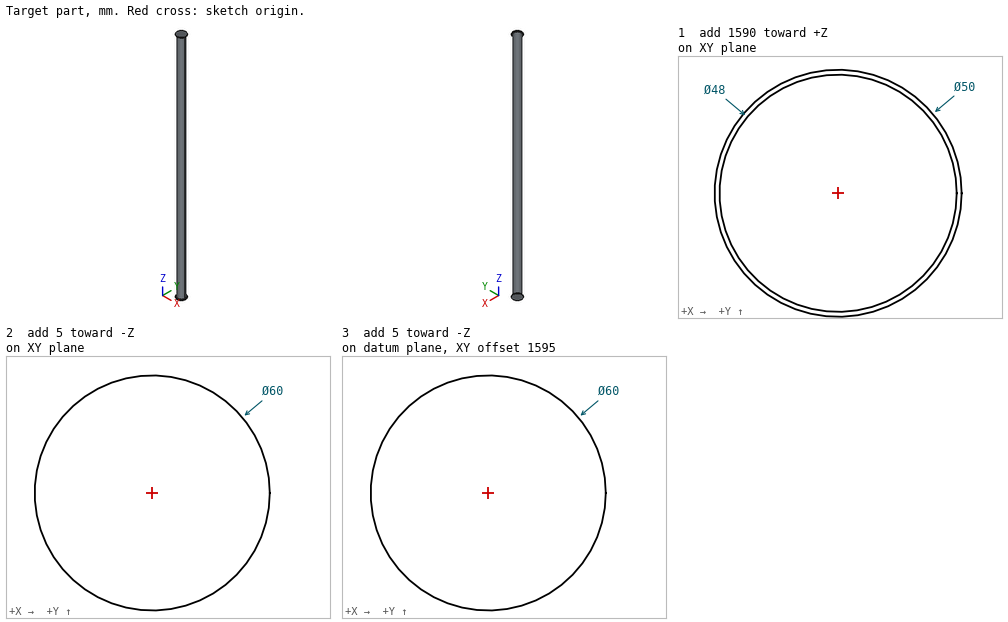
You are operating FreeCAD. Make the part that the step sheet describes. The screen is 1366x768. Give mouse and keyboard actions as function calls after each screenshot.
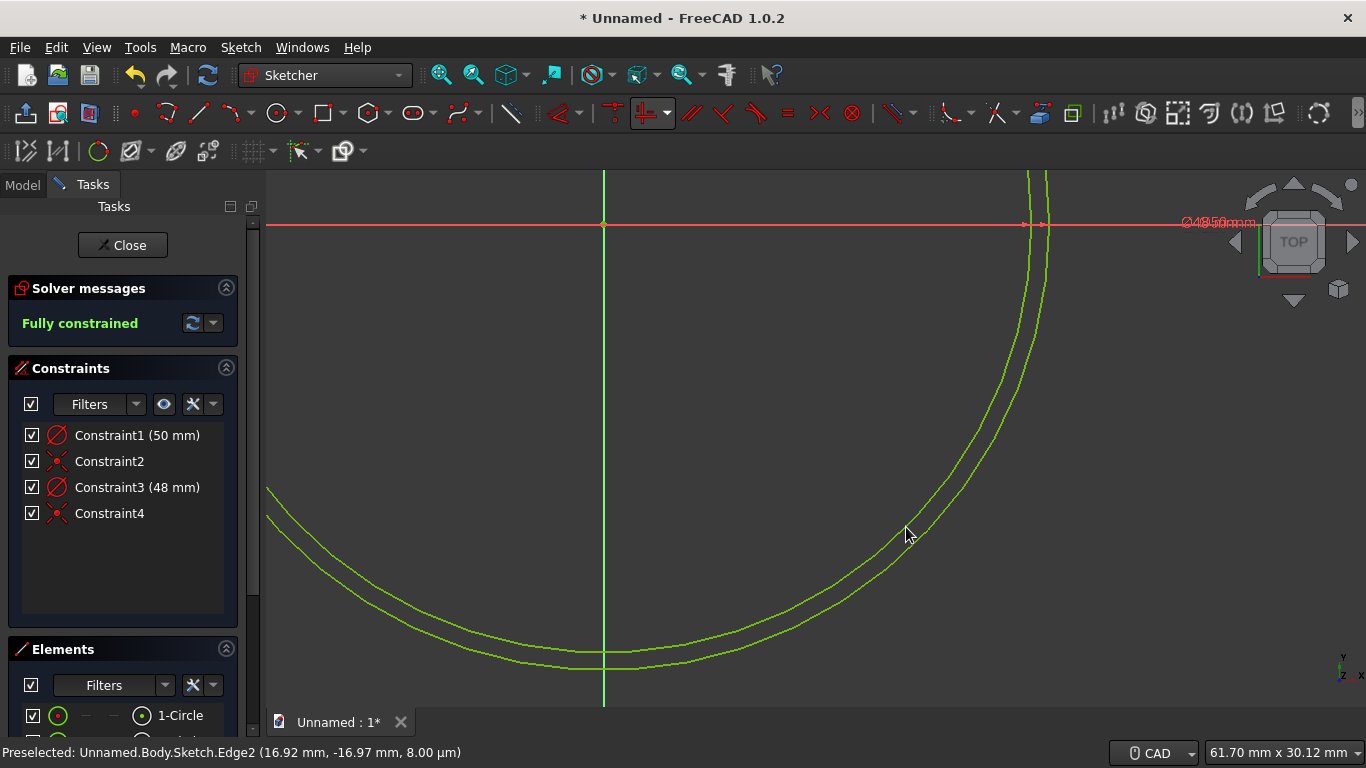
click(123, 245)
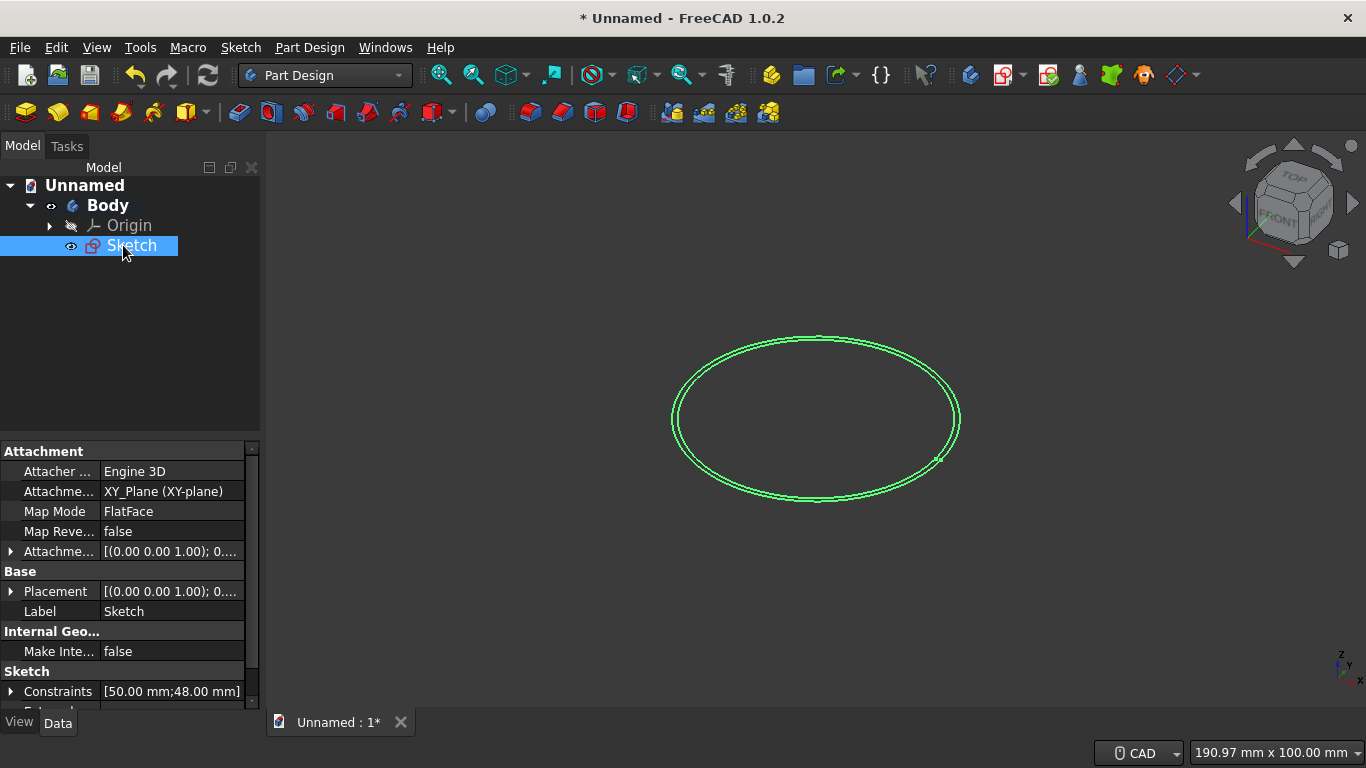
click(26, 112)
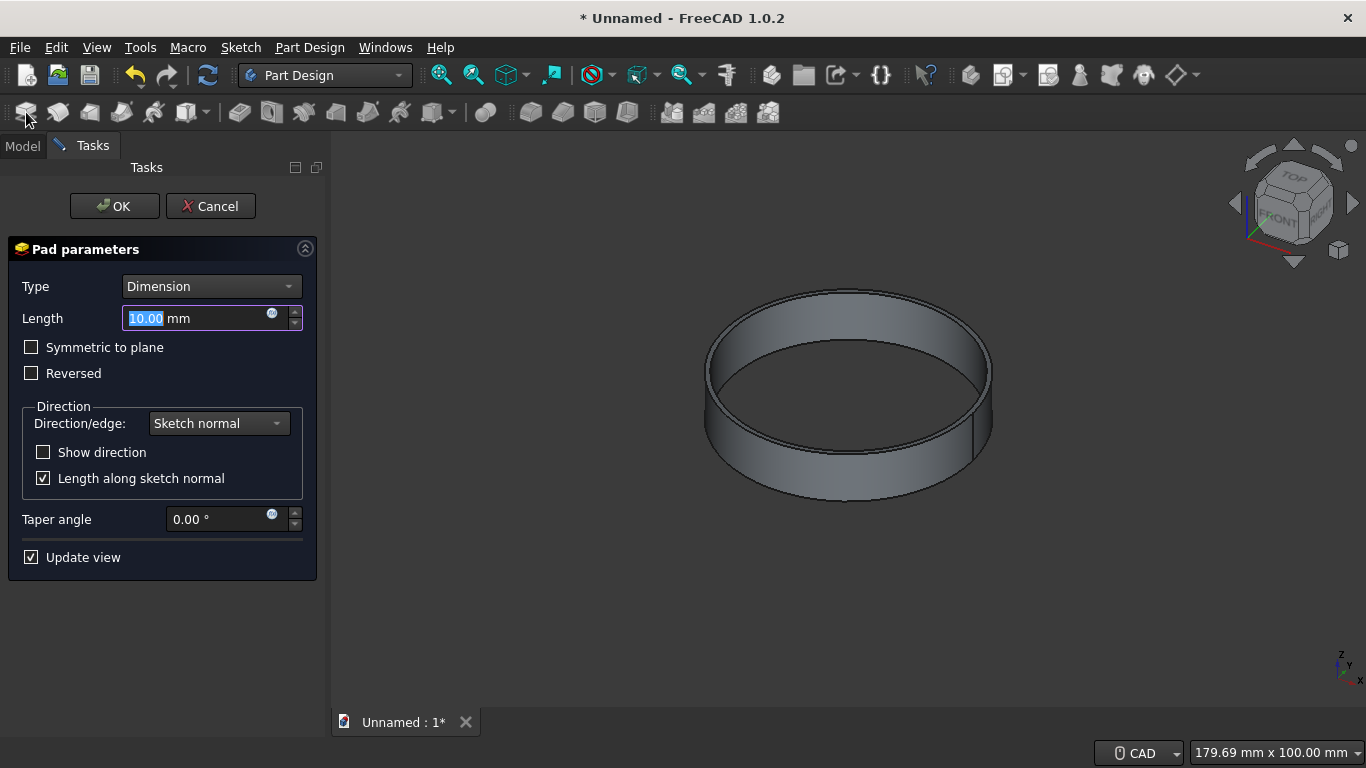
text(1590)
key(Tab)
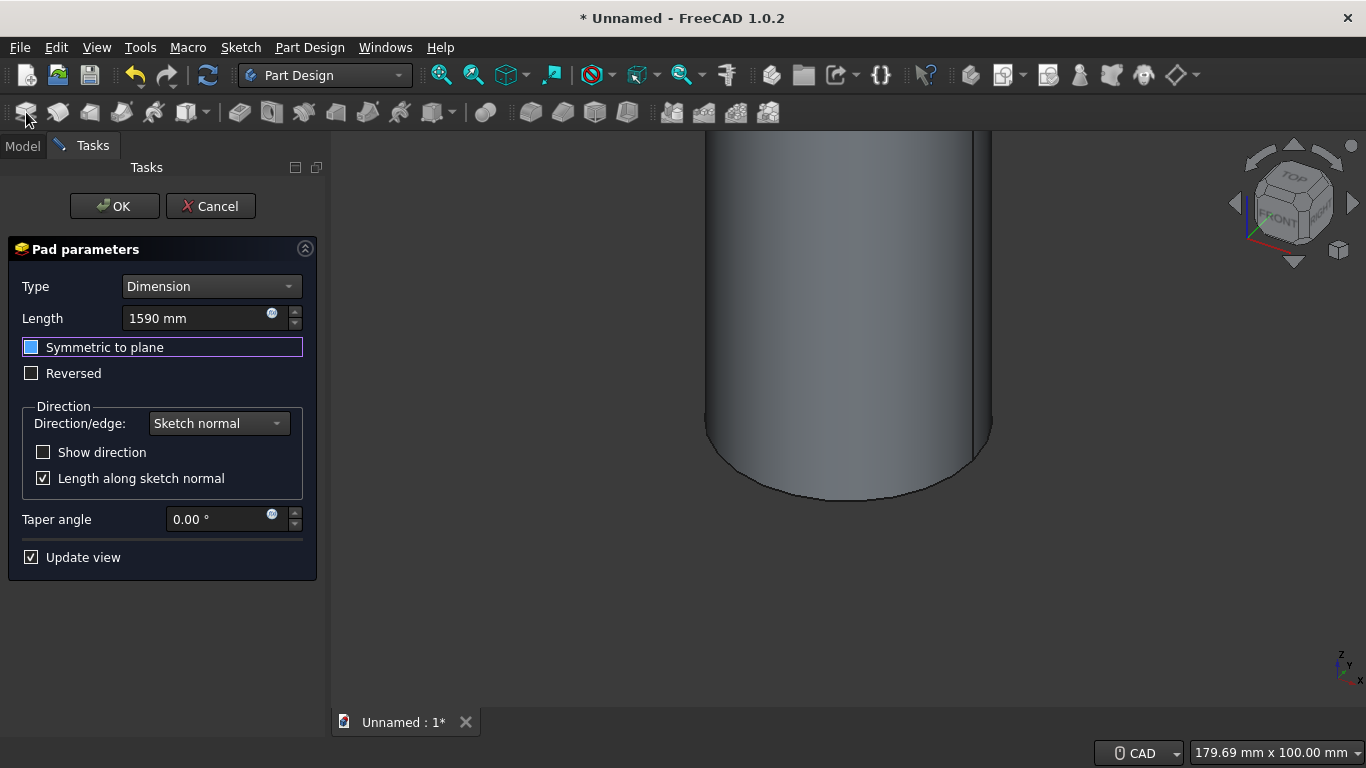
click(115, 206)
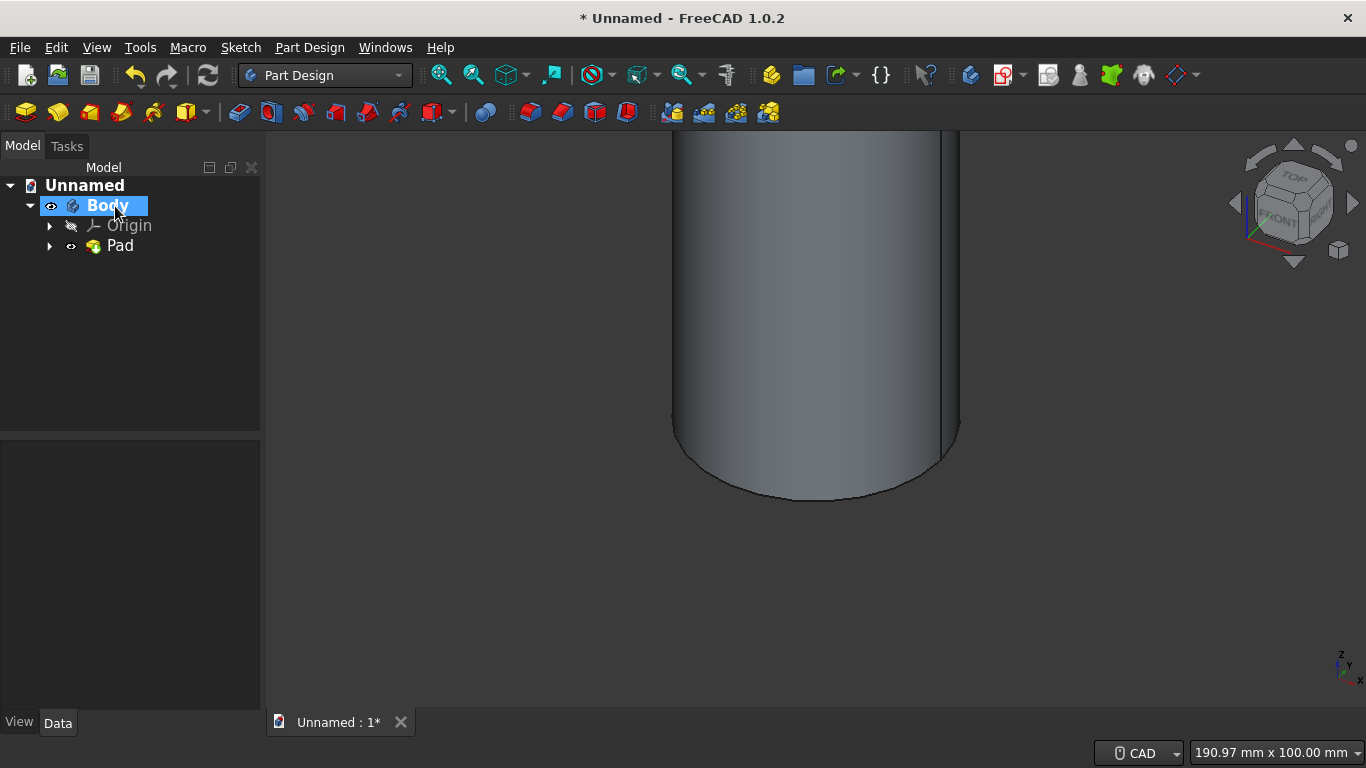
click(442, 76)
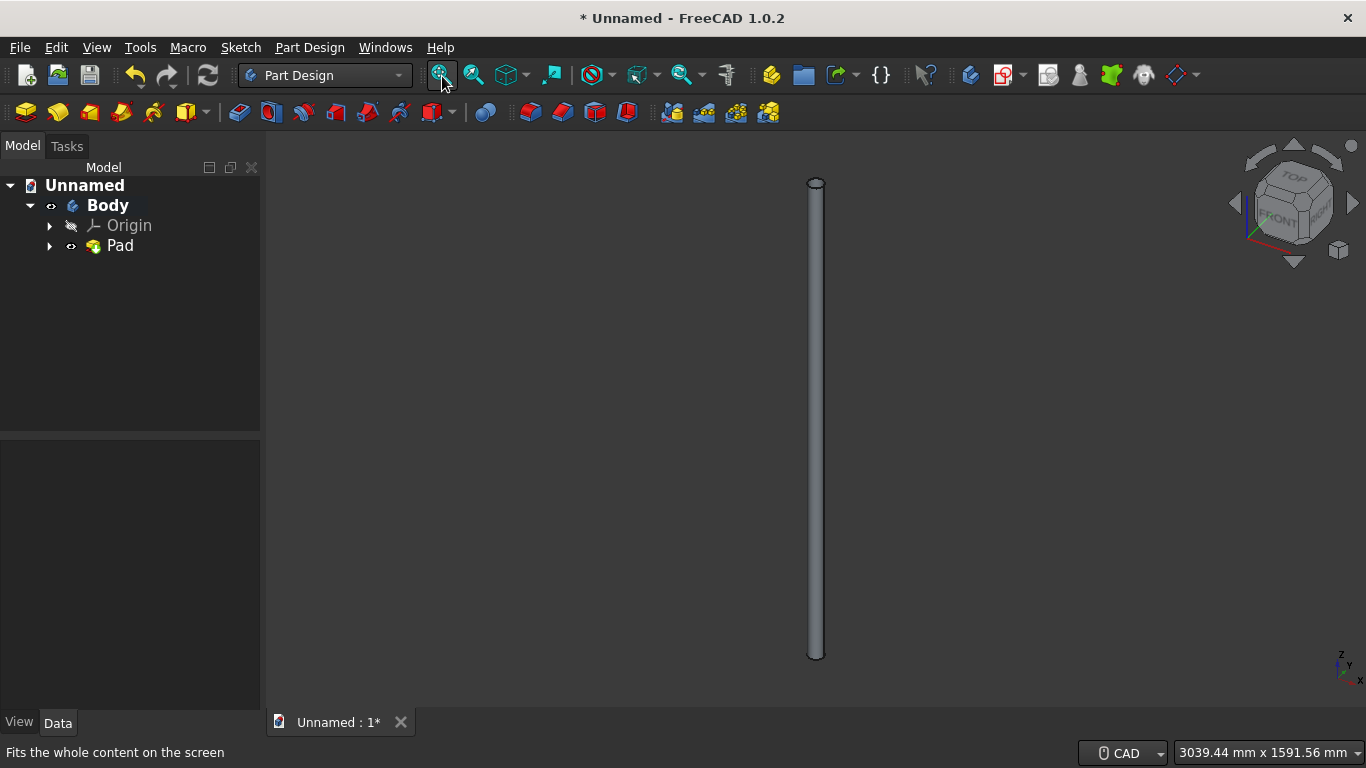
click(1004, 76)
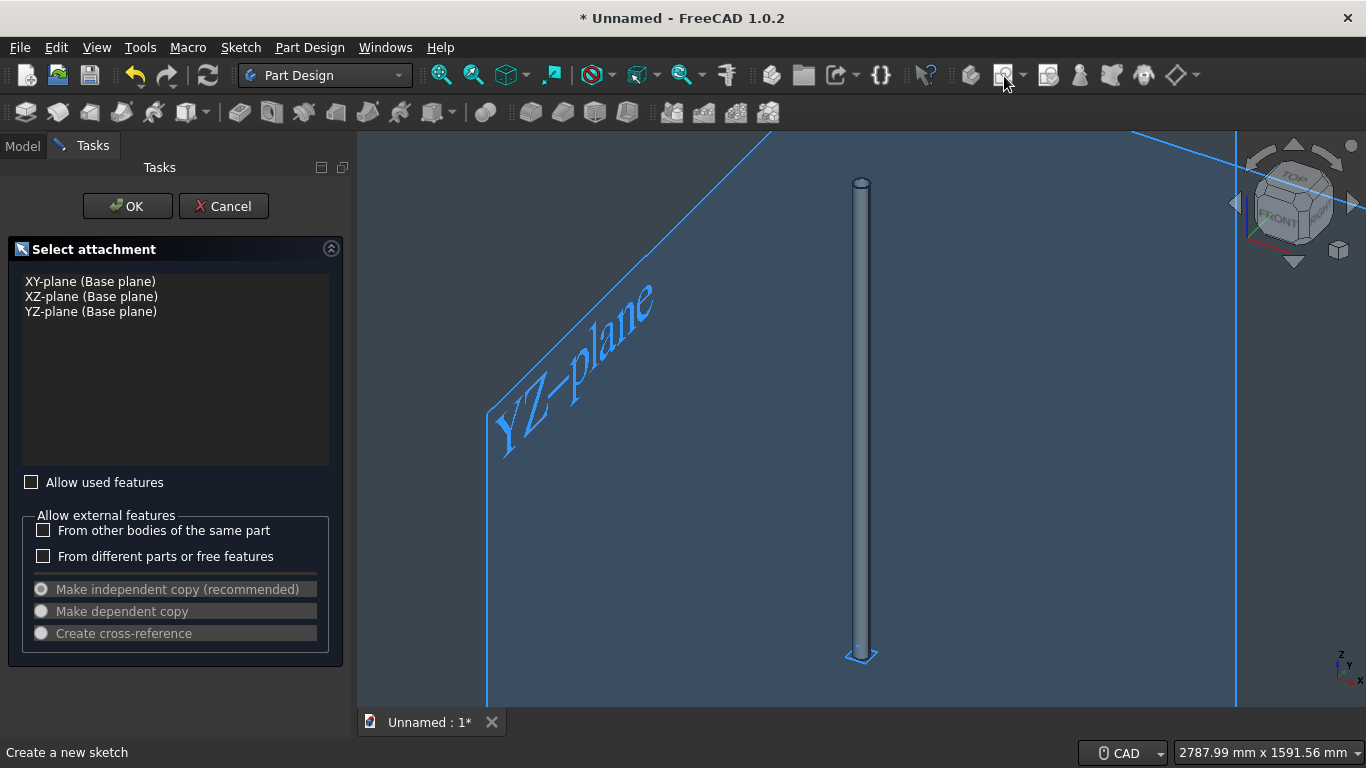
click(82, 282)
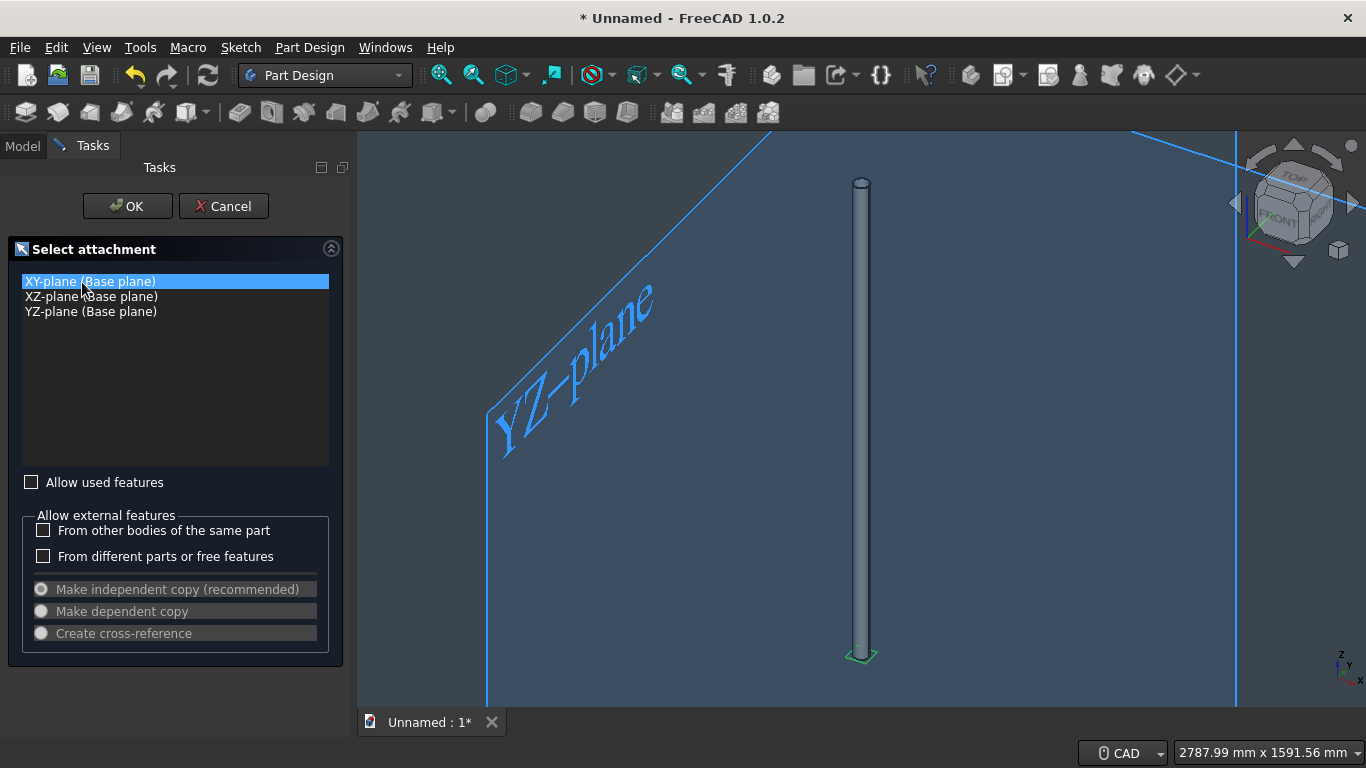
click(128, 206)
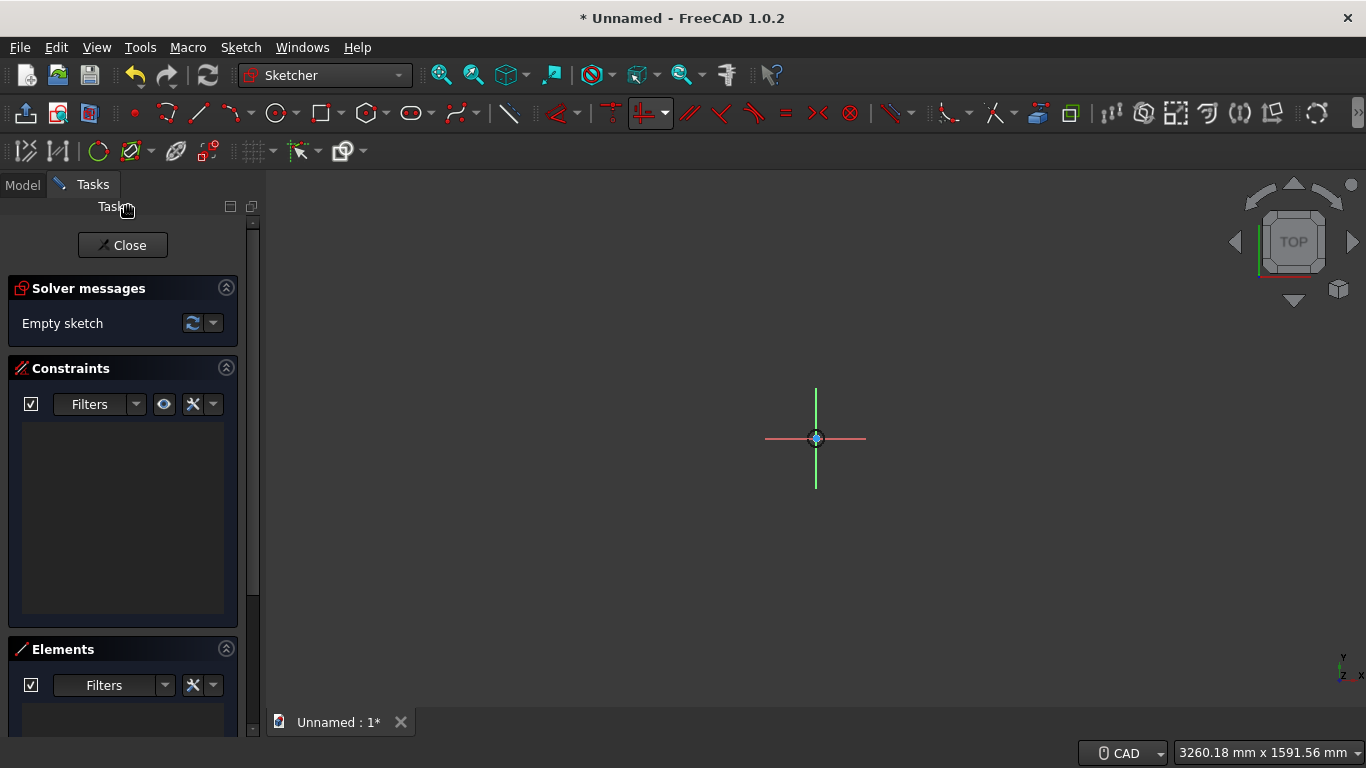
click(90, 114)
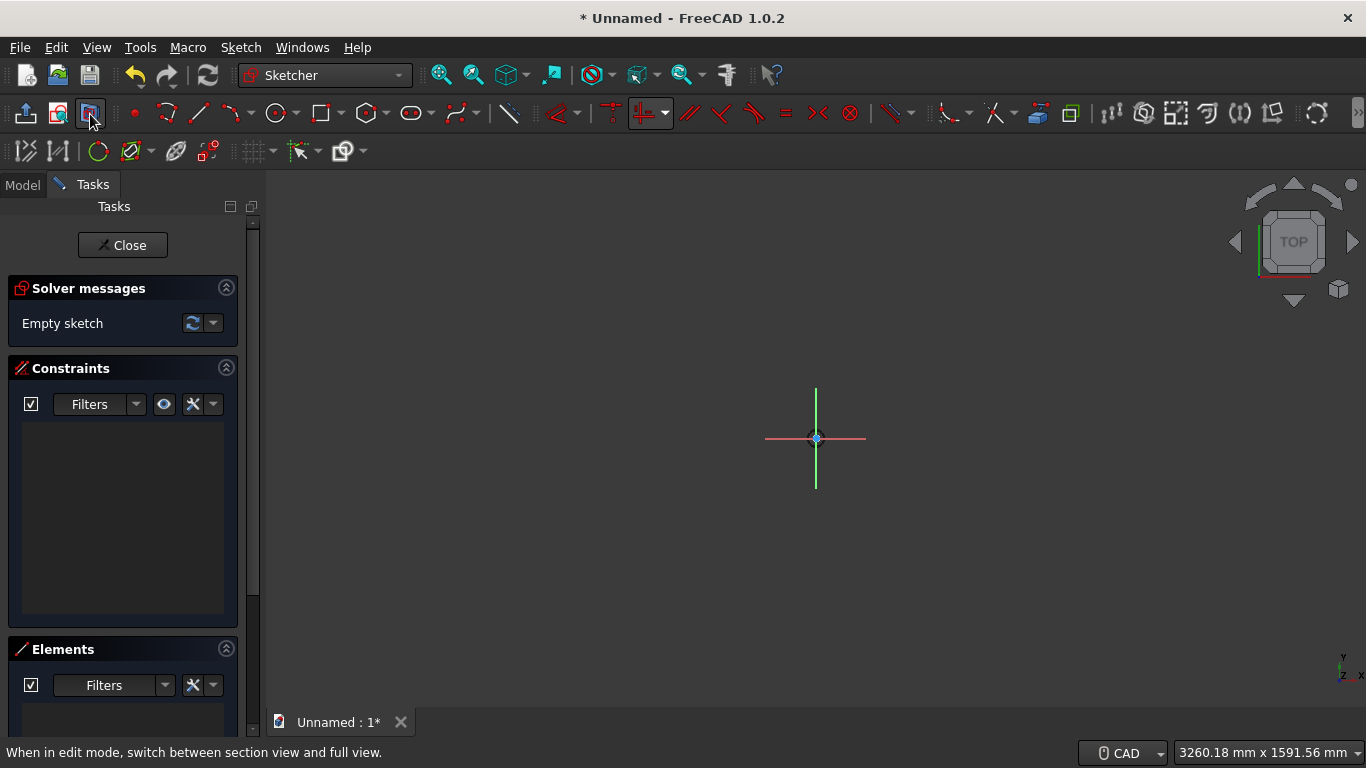
scroll(820, 438, up, 14)